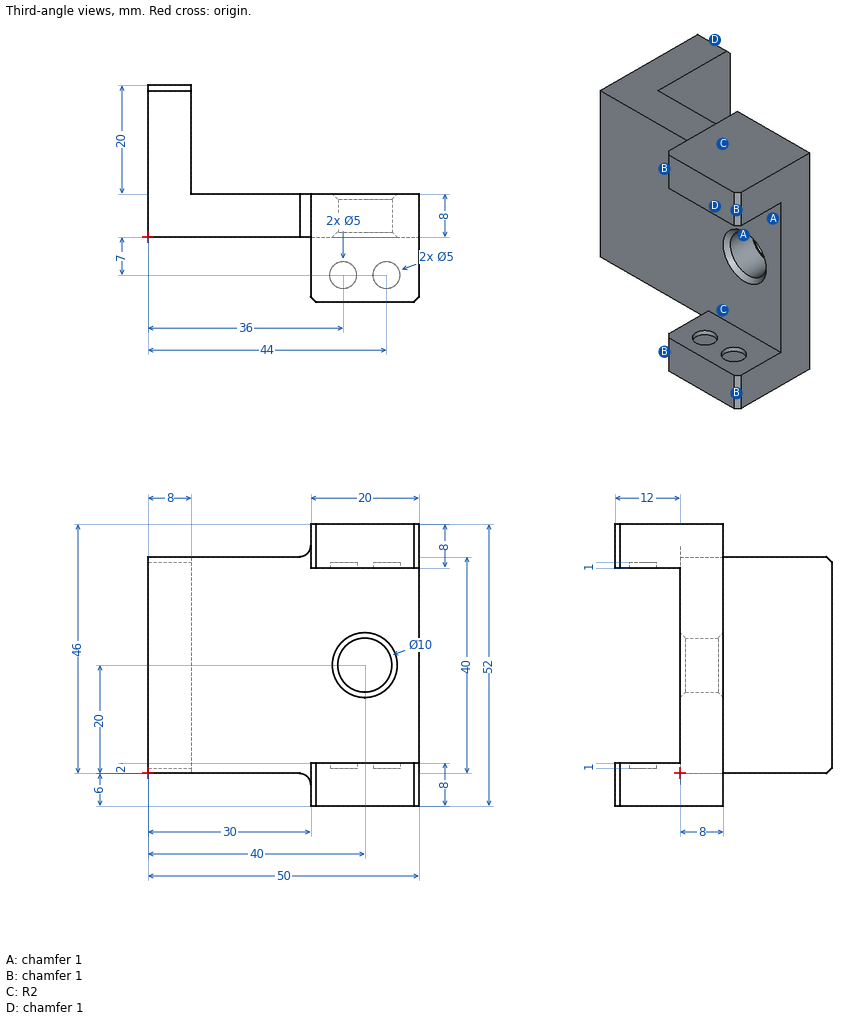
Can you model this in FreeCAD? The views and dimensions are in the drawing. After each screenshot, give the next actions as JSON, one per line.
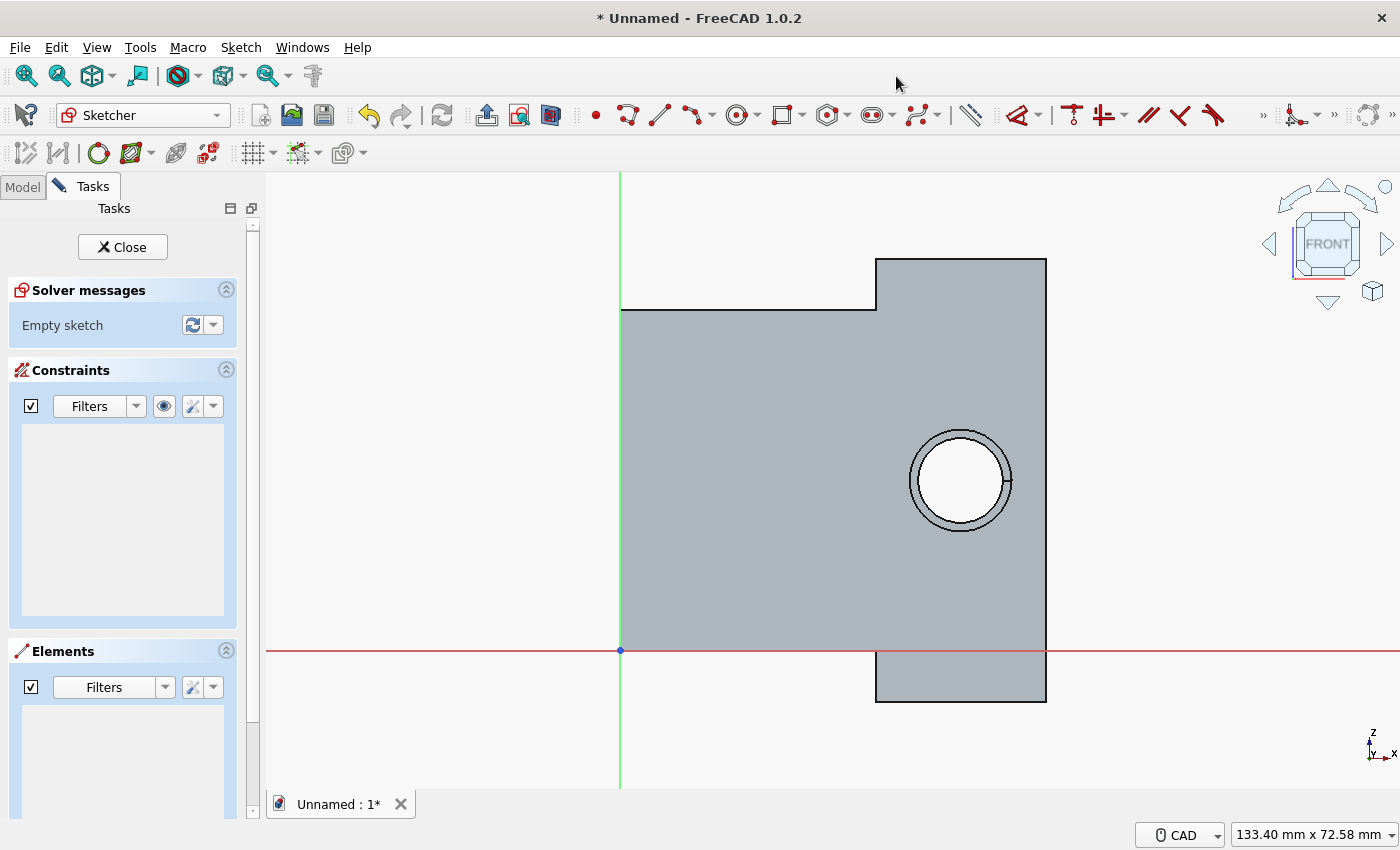
{"action": "left_click", "coordinate": [782, 116]}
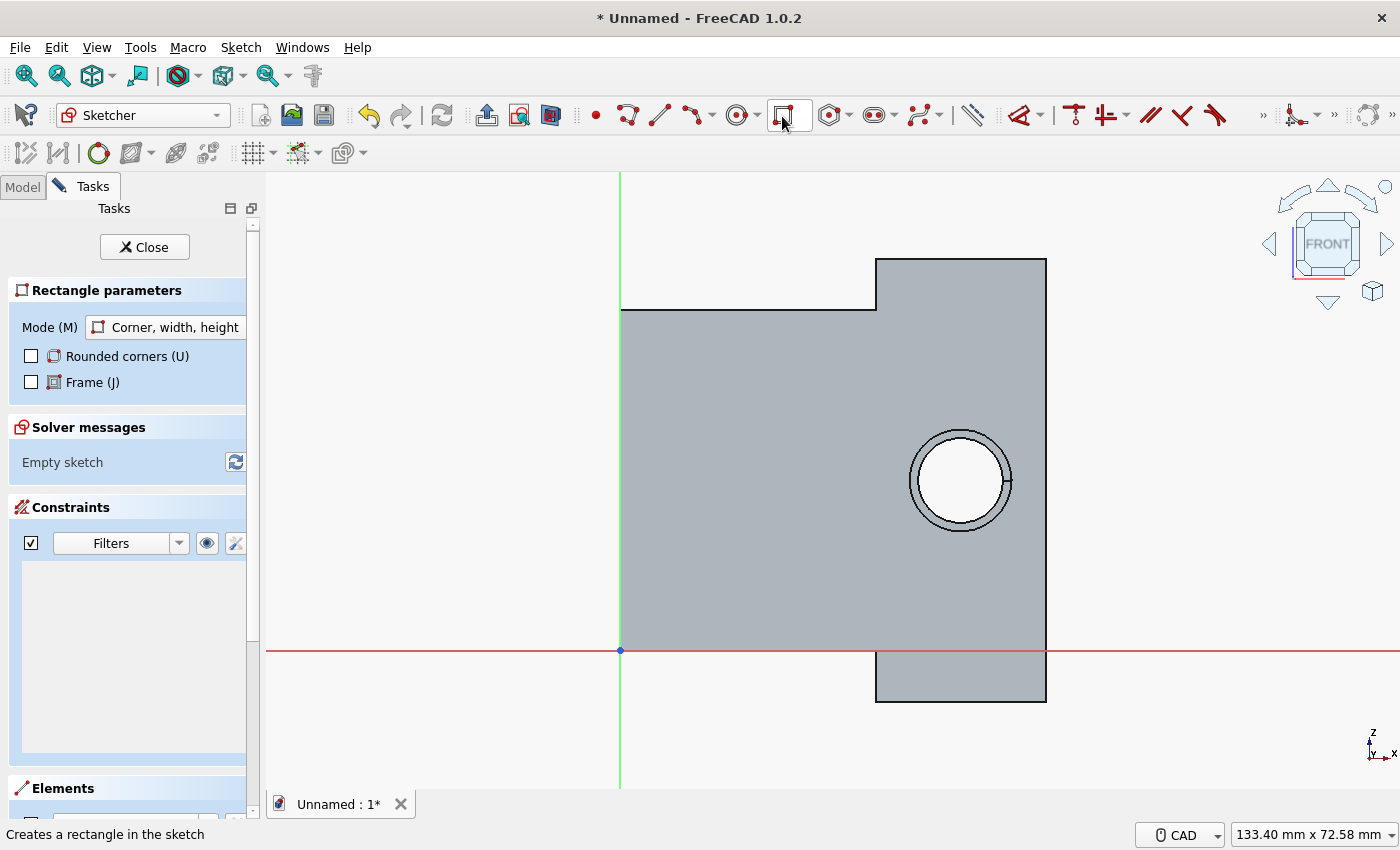
{"action": "left_click", "coordinate": [876, 259]}
{"action": "mouse_move", "coordinate": [1046, 327]}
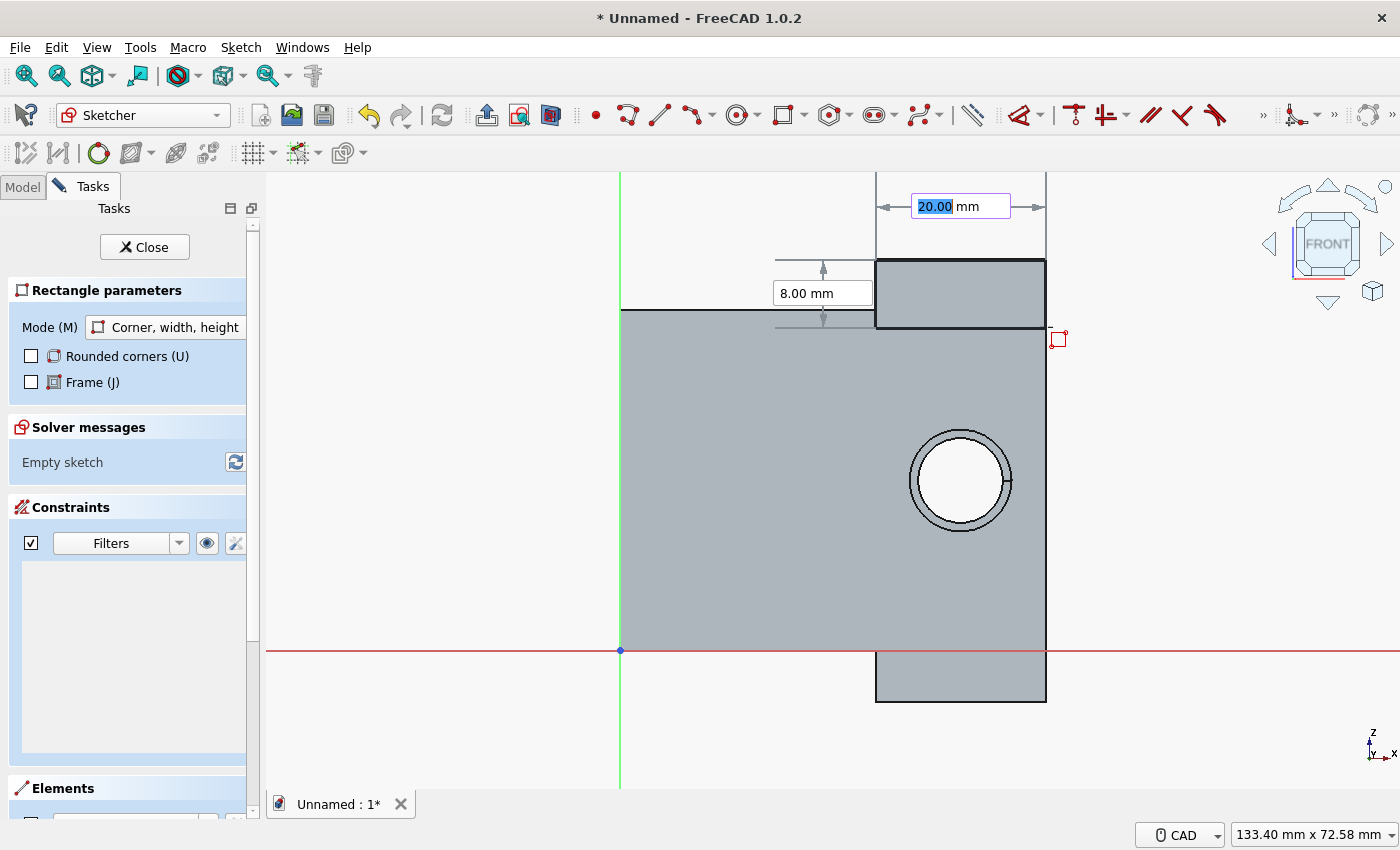
{"action": "type", "text": "20"}
{"action": "key", "text": "Tab"}
{"action": "type", "text": "8"}
{"action": "key", "text": "Return"}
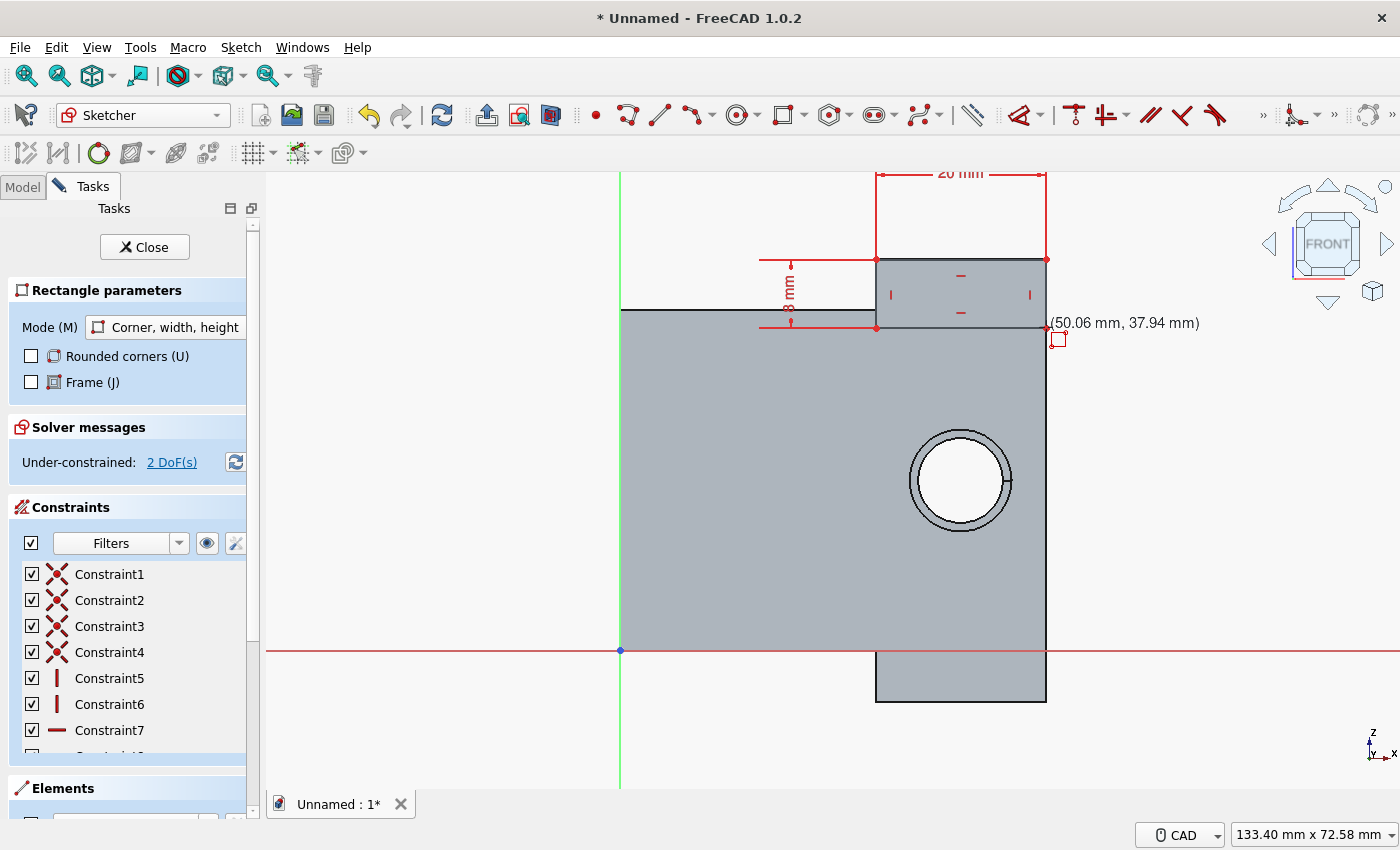
{"action": "left_click", "coordinate": [876, 634]}
{"action": "mouse_move", "coordinate": [1046, 702]}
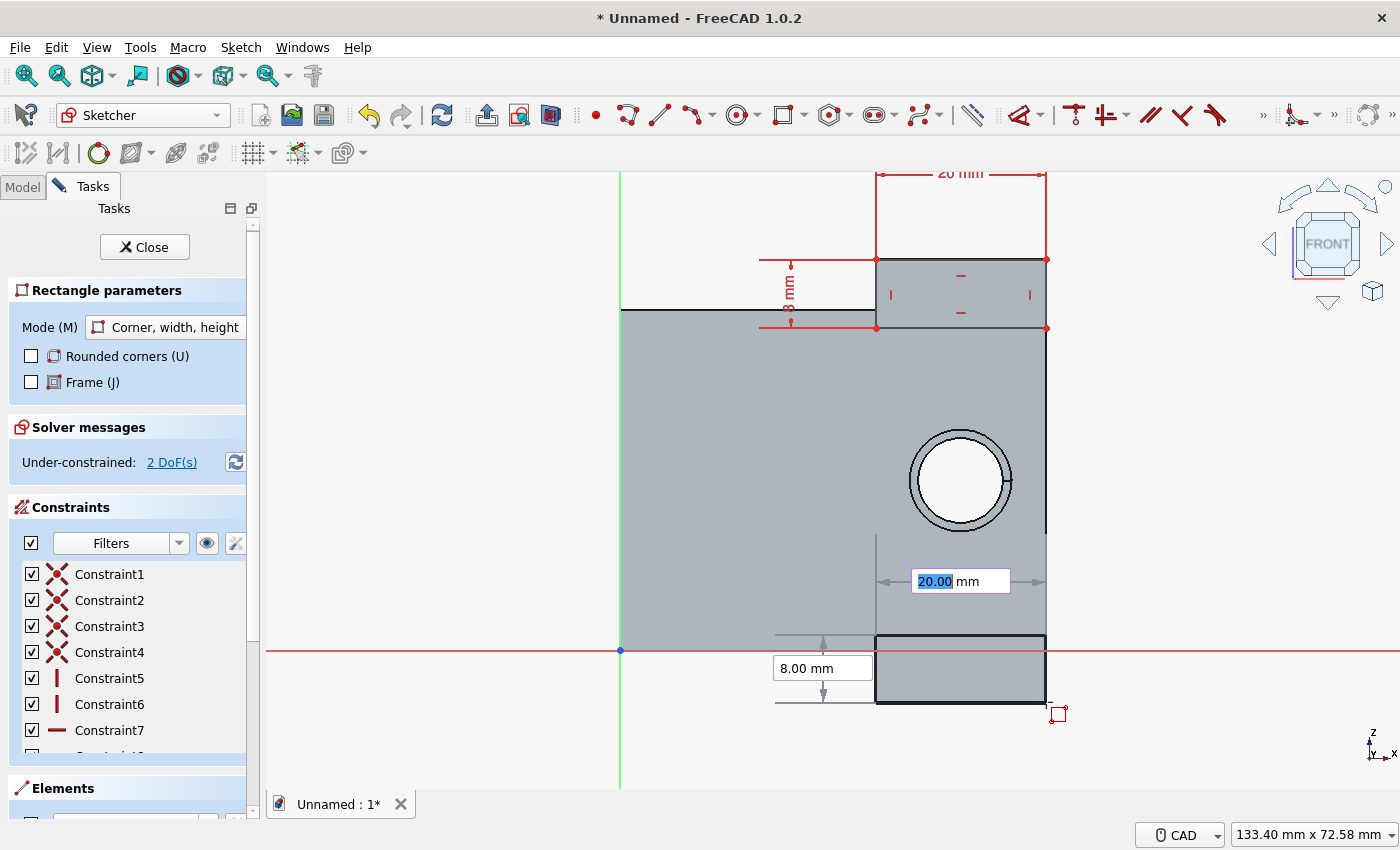
{"action": "type", "text": "20"}
{"action": "key", "text": "Tab"}
{"action": "type", "text": "8"}
{"action": "key", "text": "Return"}
{"action": "key", "text": "Escape"}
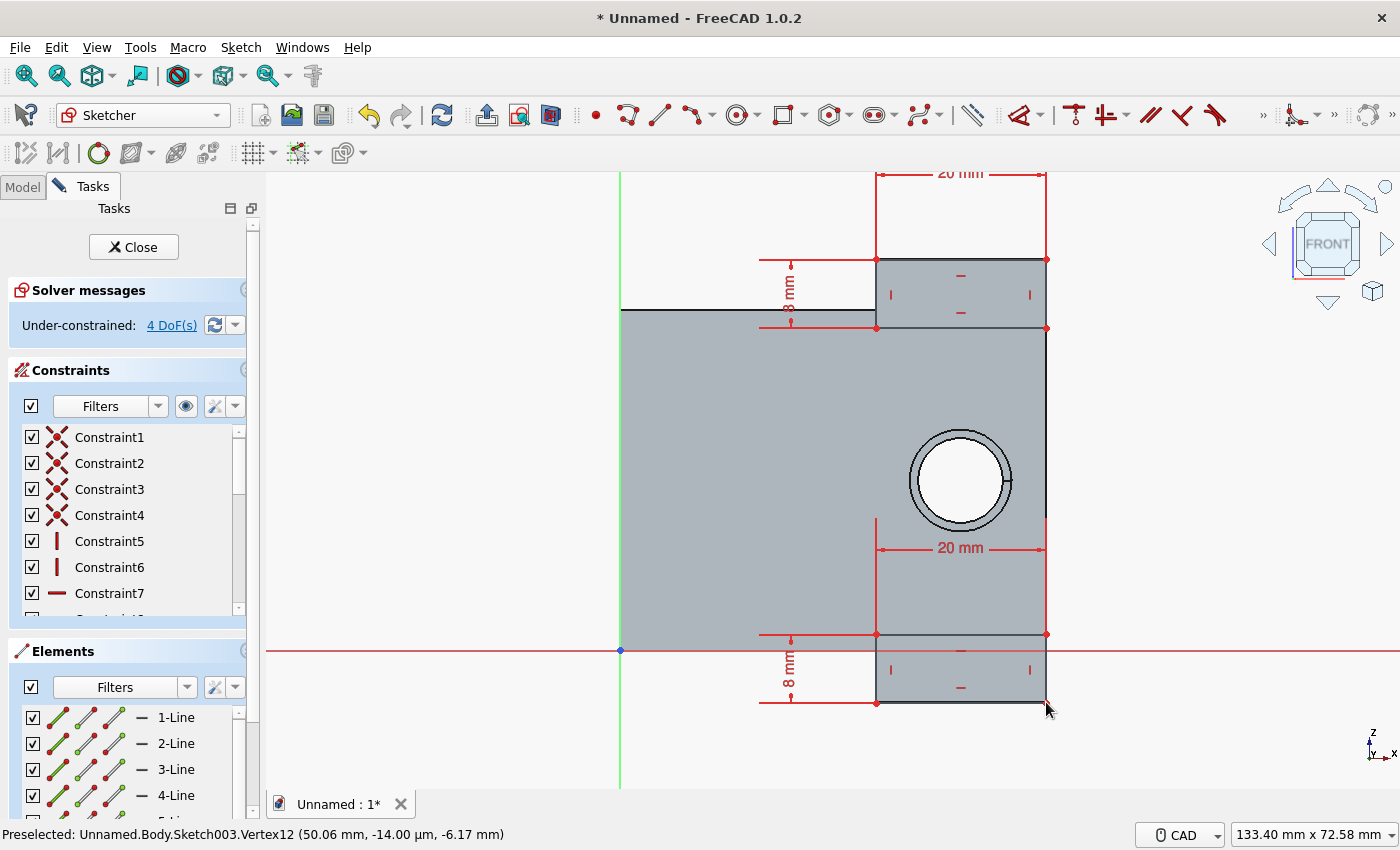
{"action": "left_click", "coordinate": [1020, 116]}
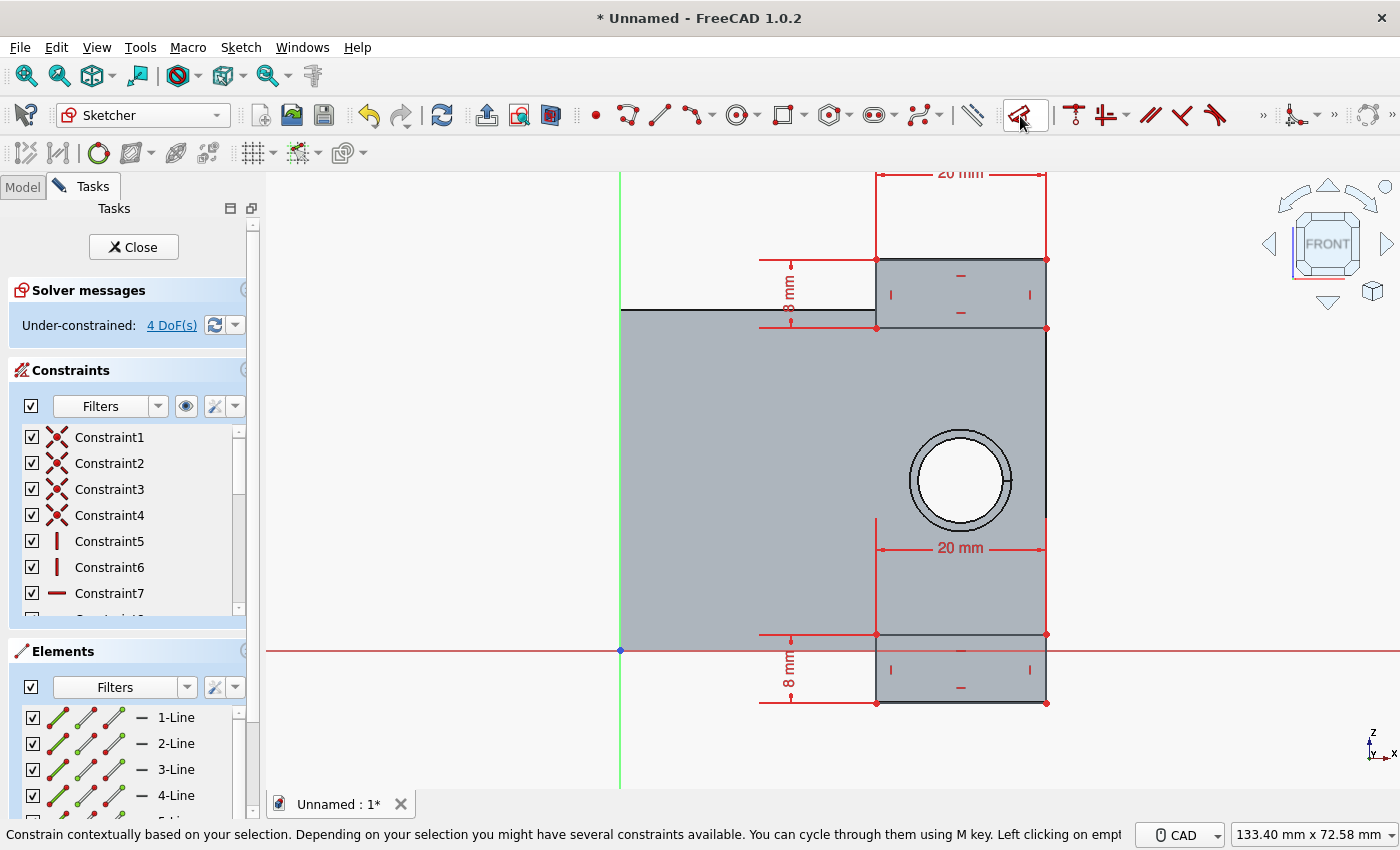
{"action": "scroll", "coordinate": [876, 635], "scroll_direction": "up", "scroll_amount": 5}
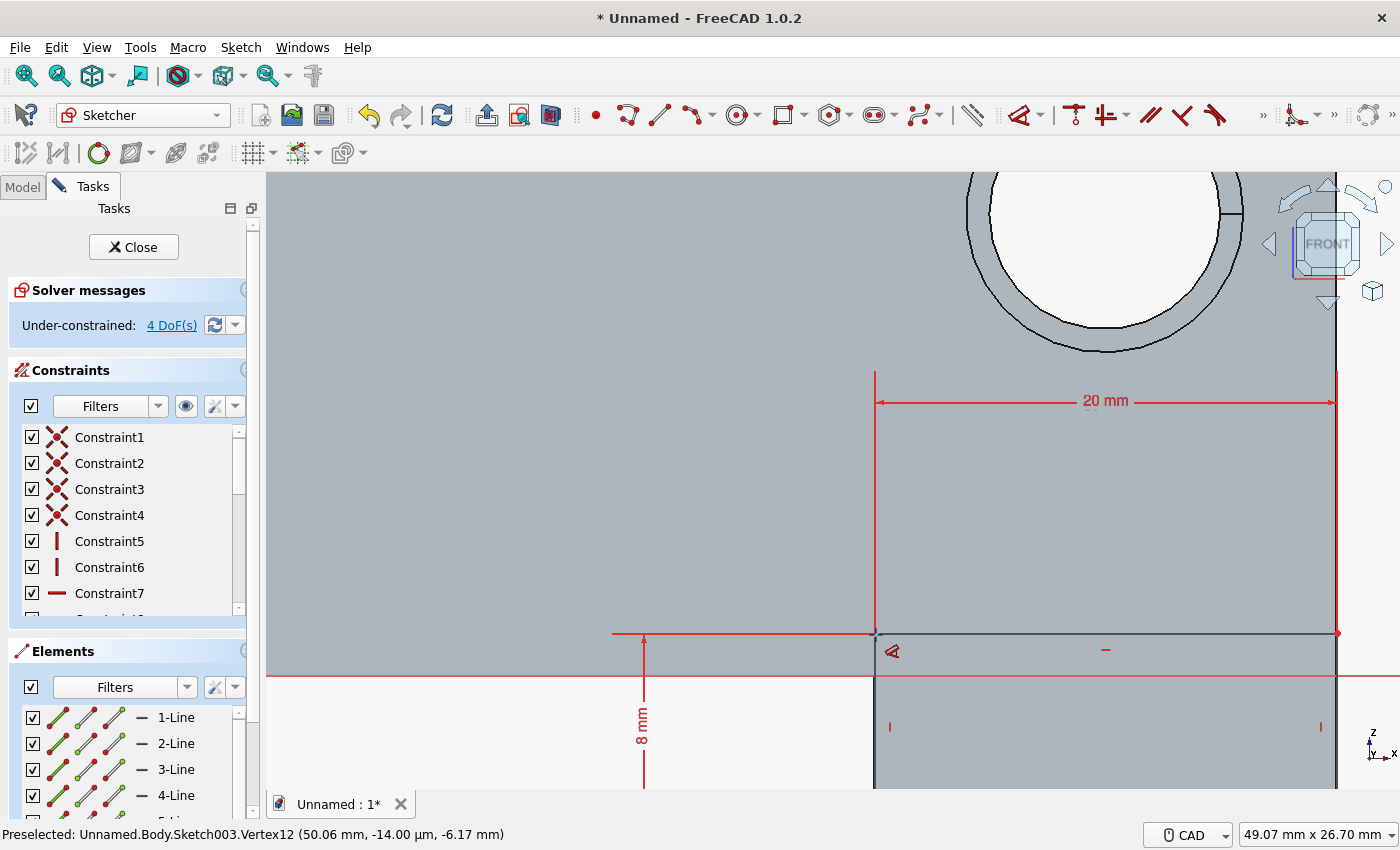
{"action": "left_click", "coordinate": [875, 634]}
{"action": "left_click", "coordinate": [909, 655]}